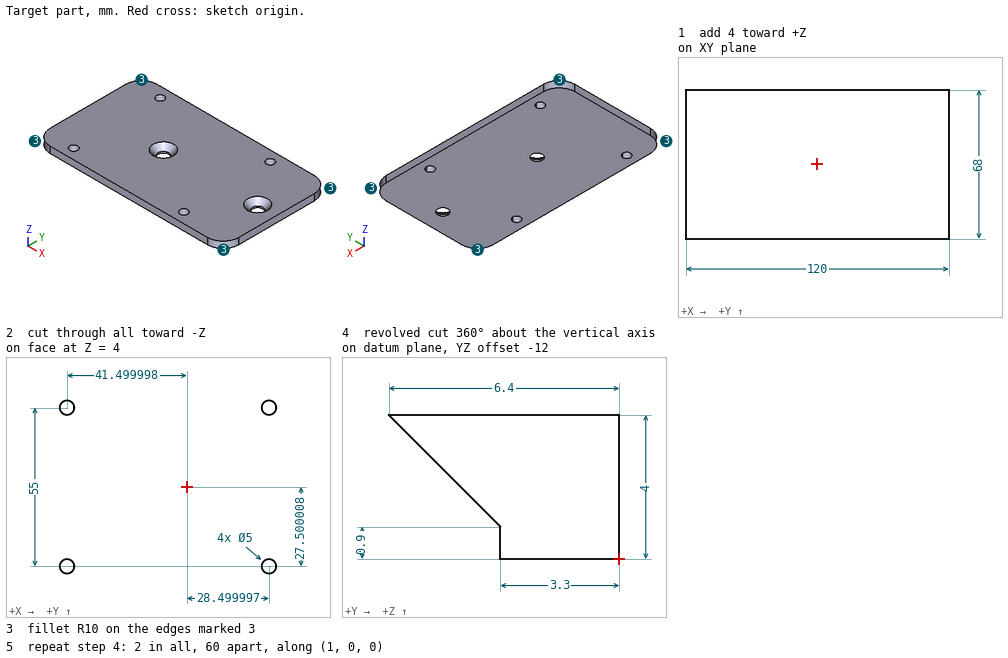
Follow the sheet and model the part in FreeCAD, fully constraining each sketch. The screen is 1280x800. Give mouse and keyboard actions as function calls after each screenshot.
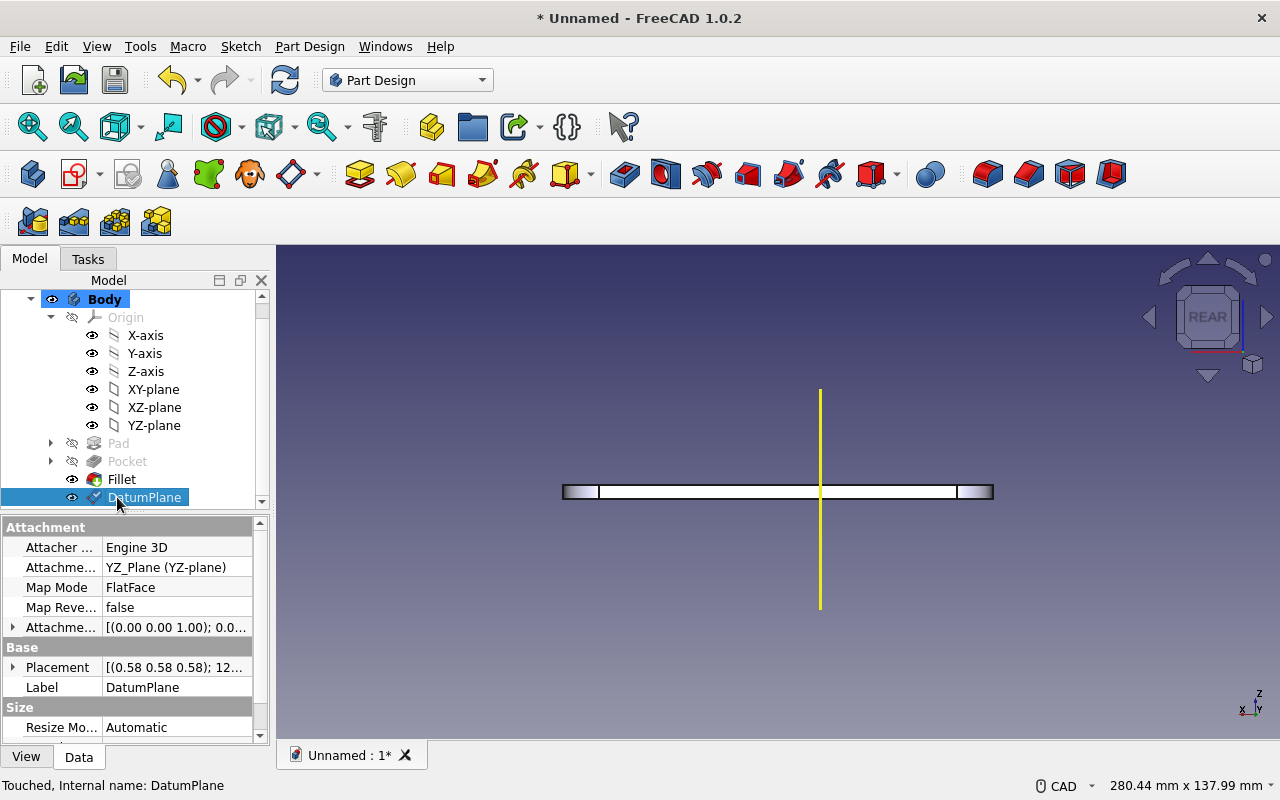
click(74, 174)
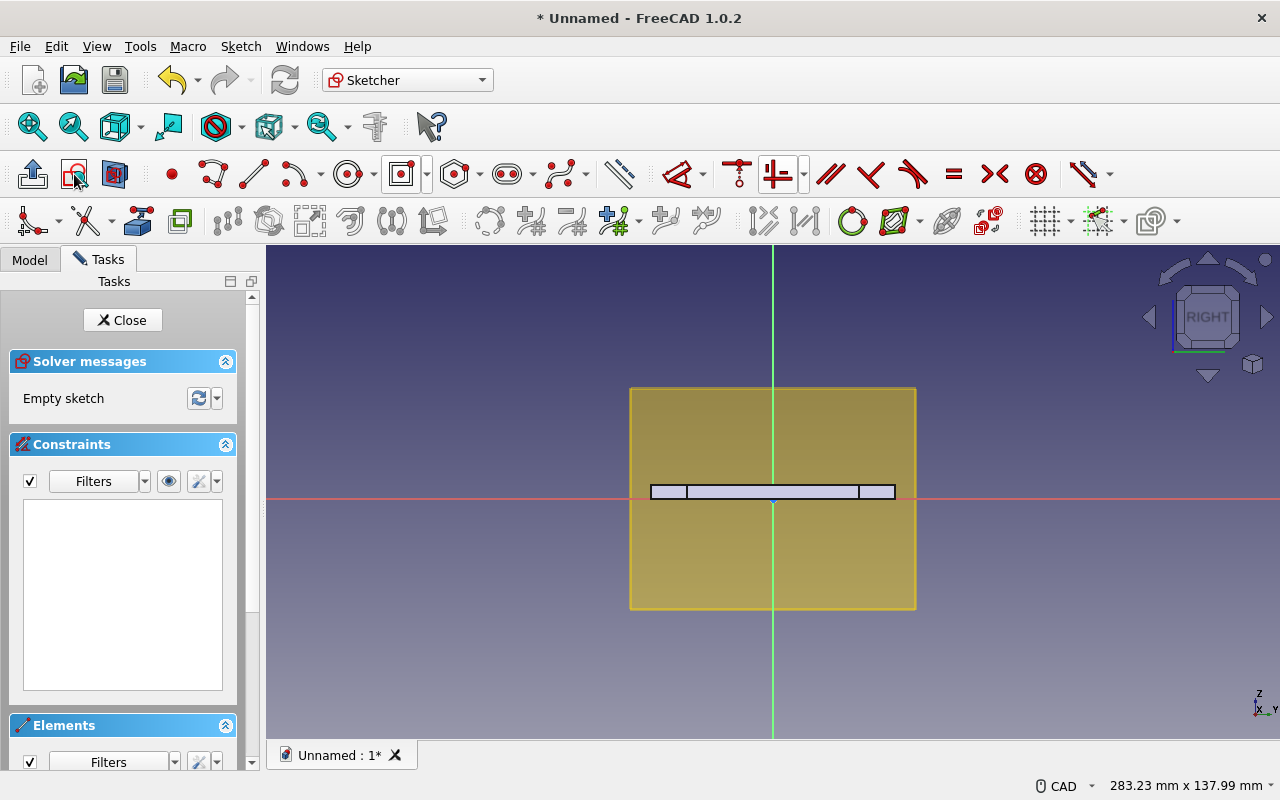
key(q)
key(s)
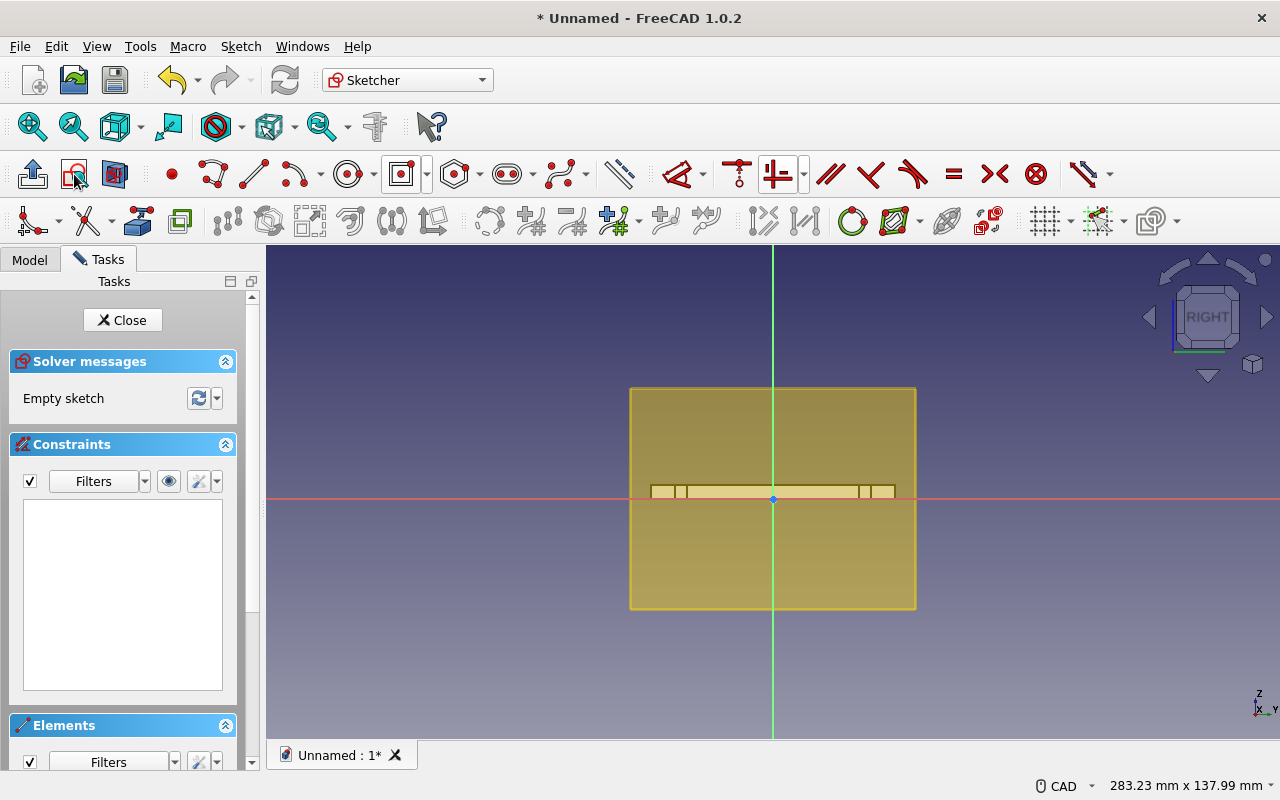
scroll(765, 492, up, 15)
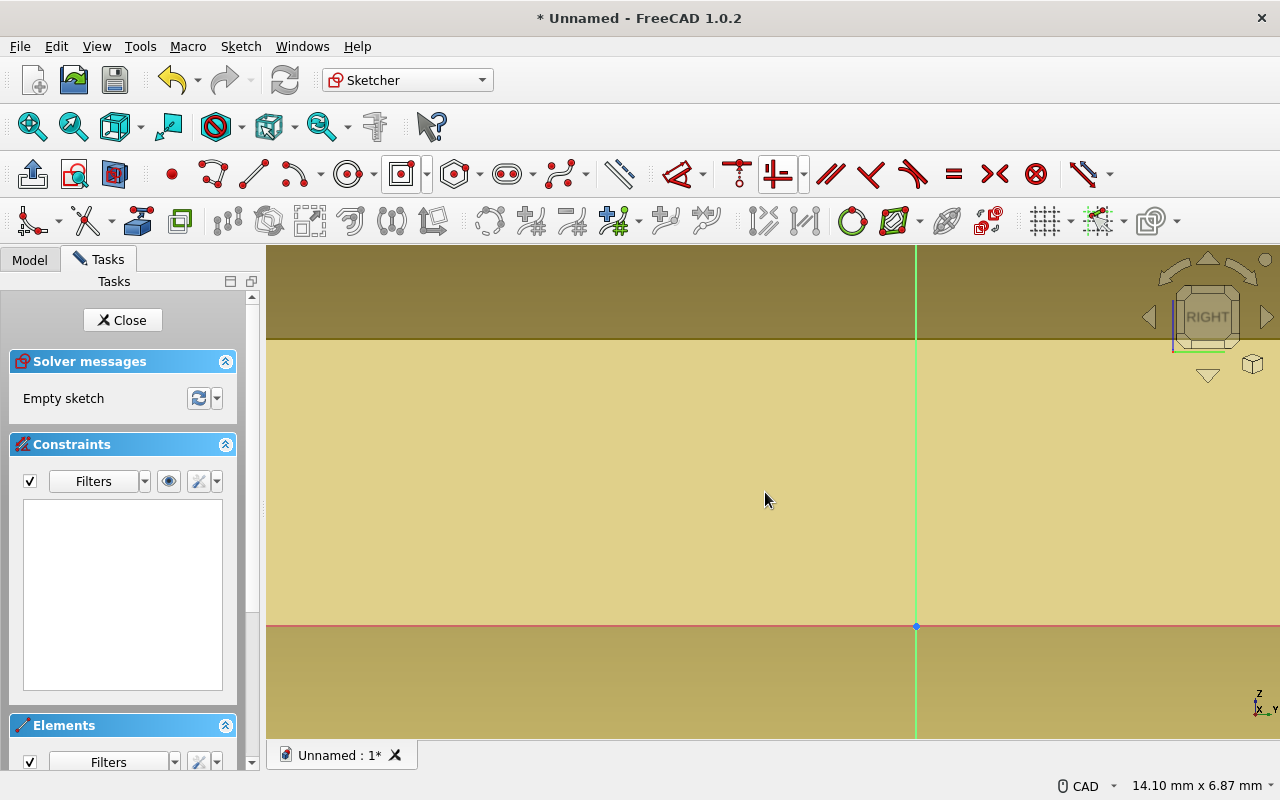
click(213, 174)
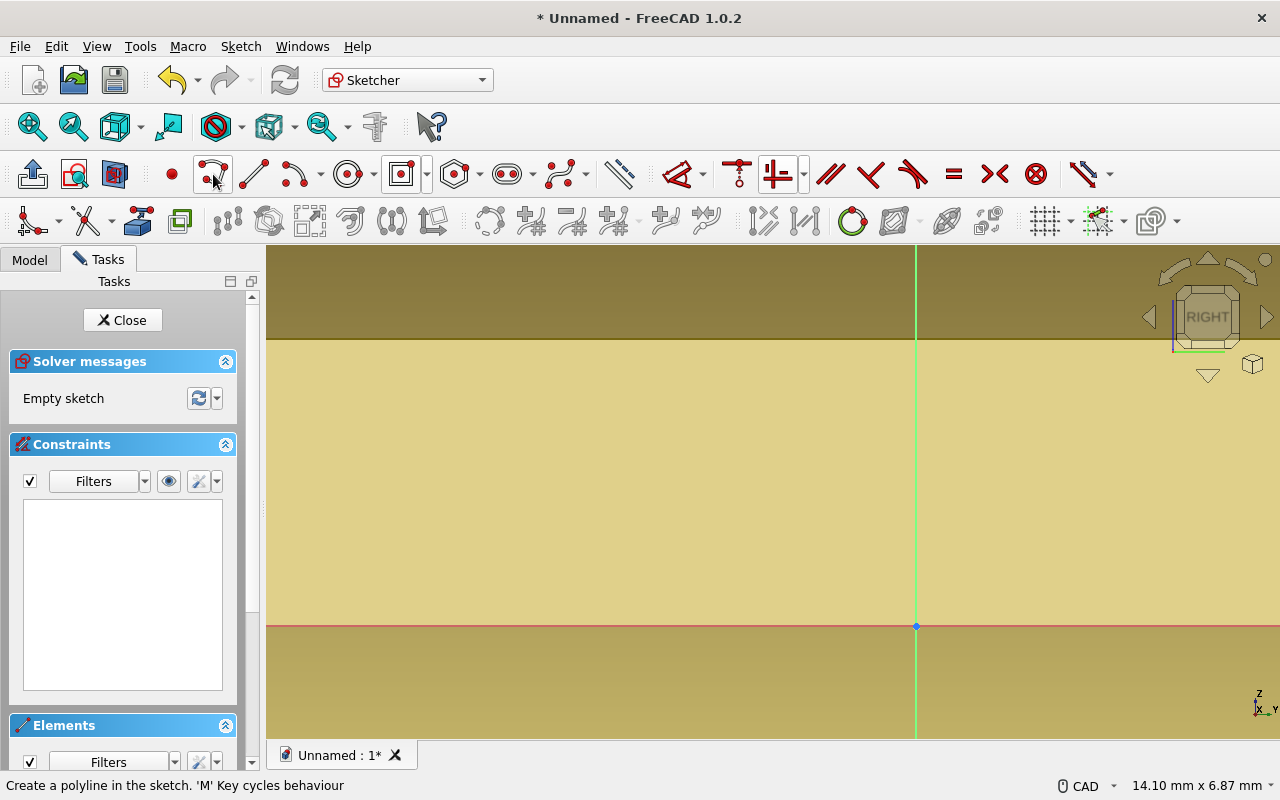
click(916, 626)
click(907, 339)
click(456, 339)
click(679, 562)
click(679, 617)
click(916, 626)
key(Escape)
key(Escape)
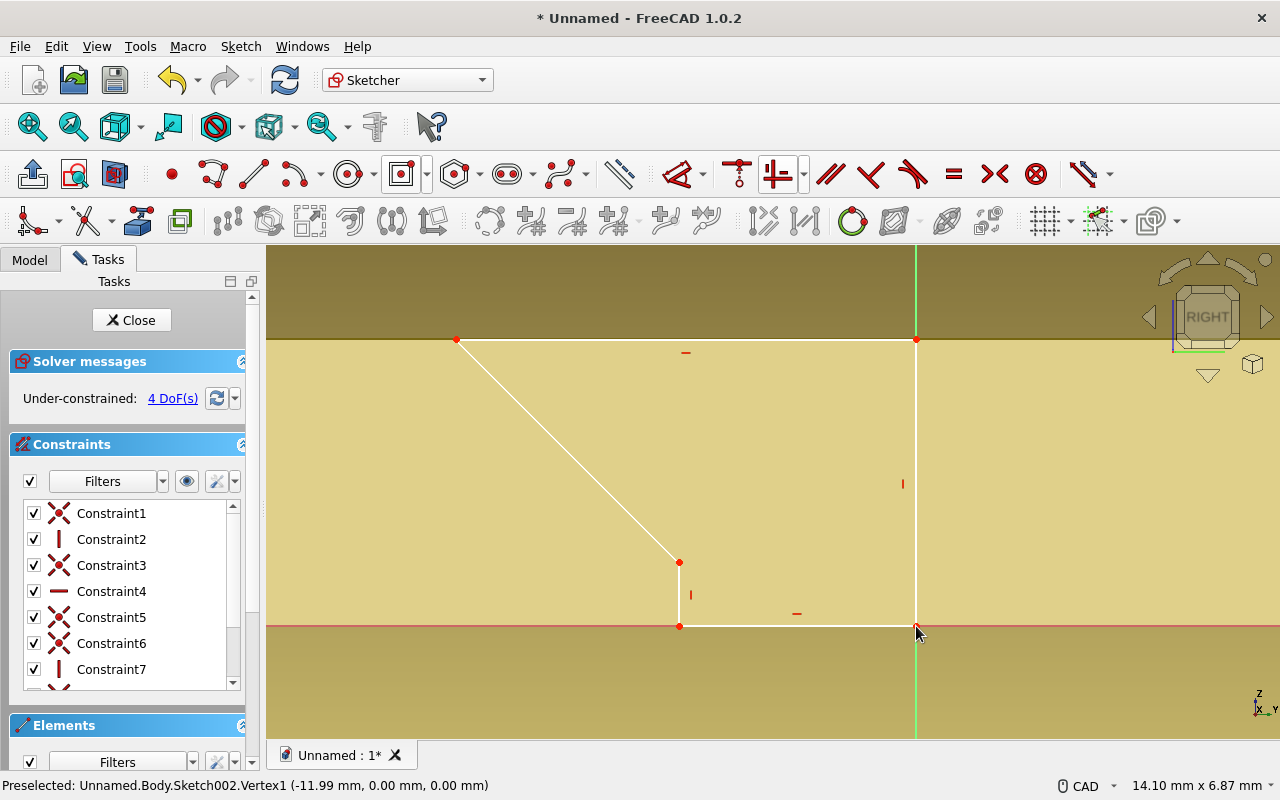
key(d)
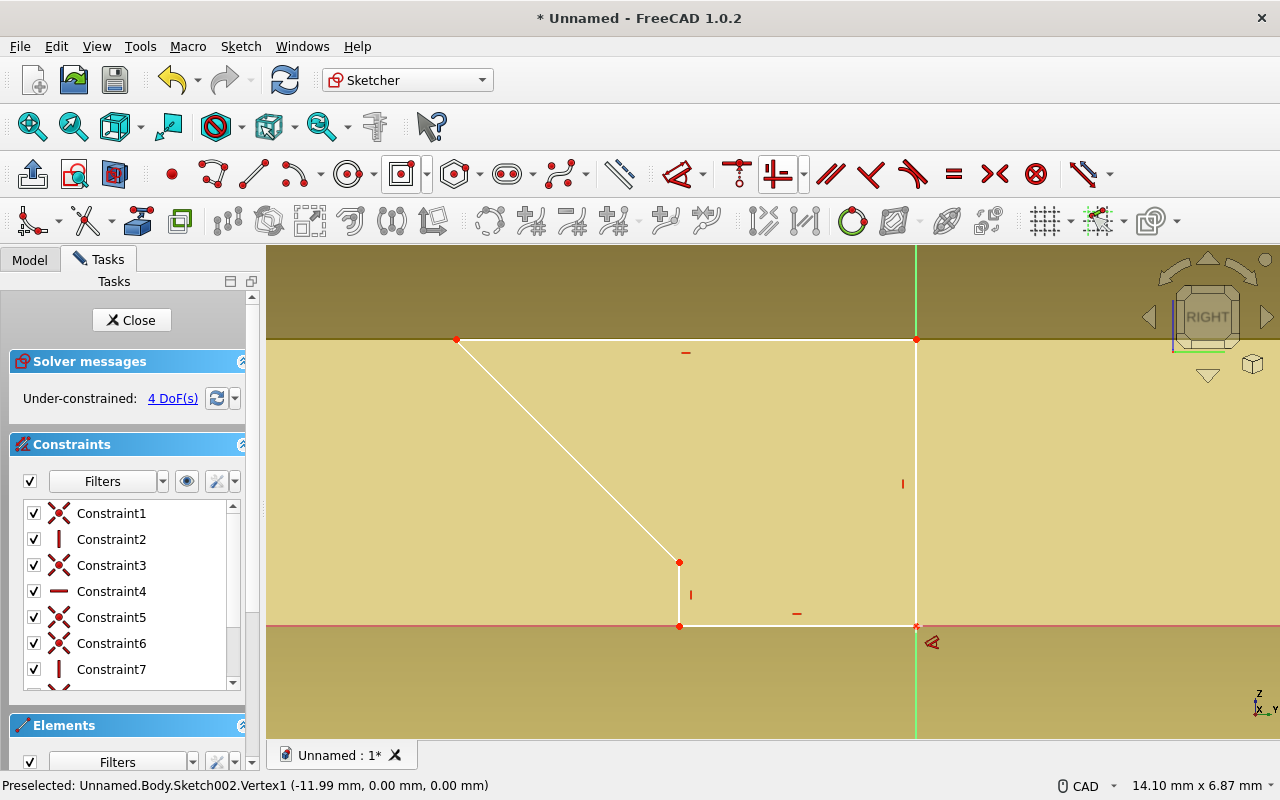
click(916, 540)
click(950, 483)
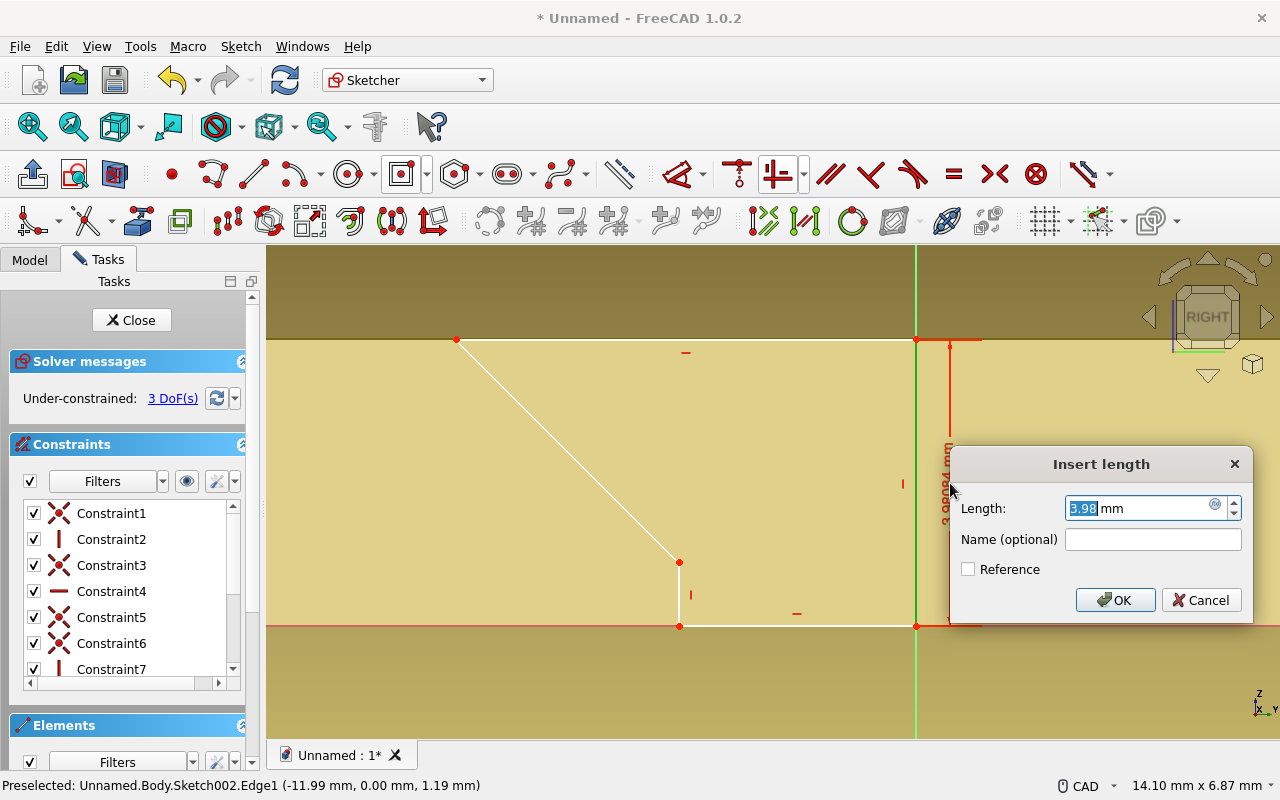
text(4)
key(Return)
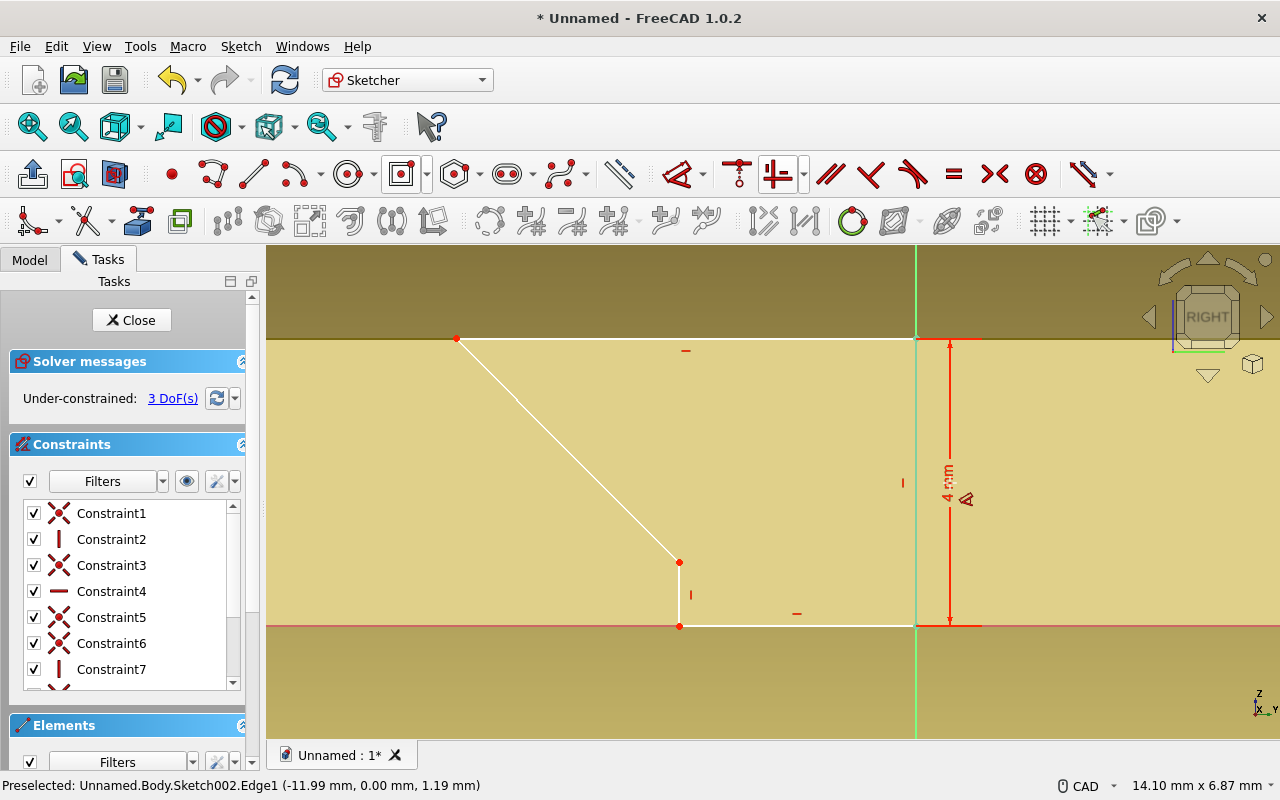
click(778, 339)
click(686, 305)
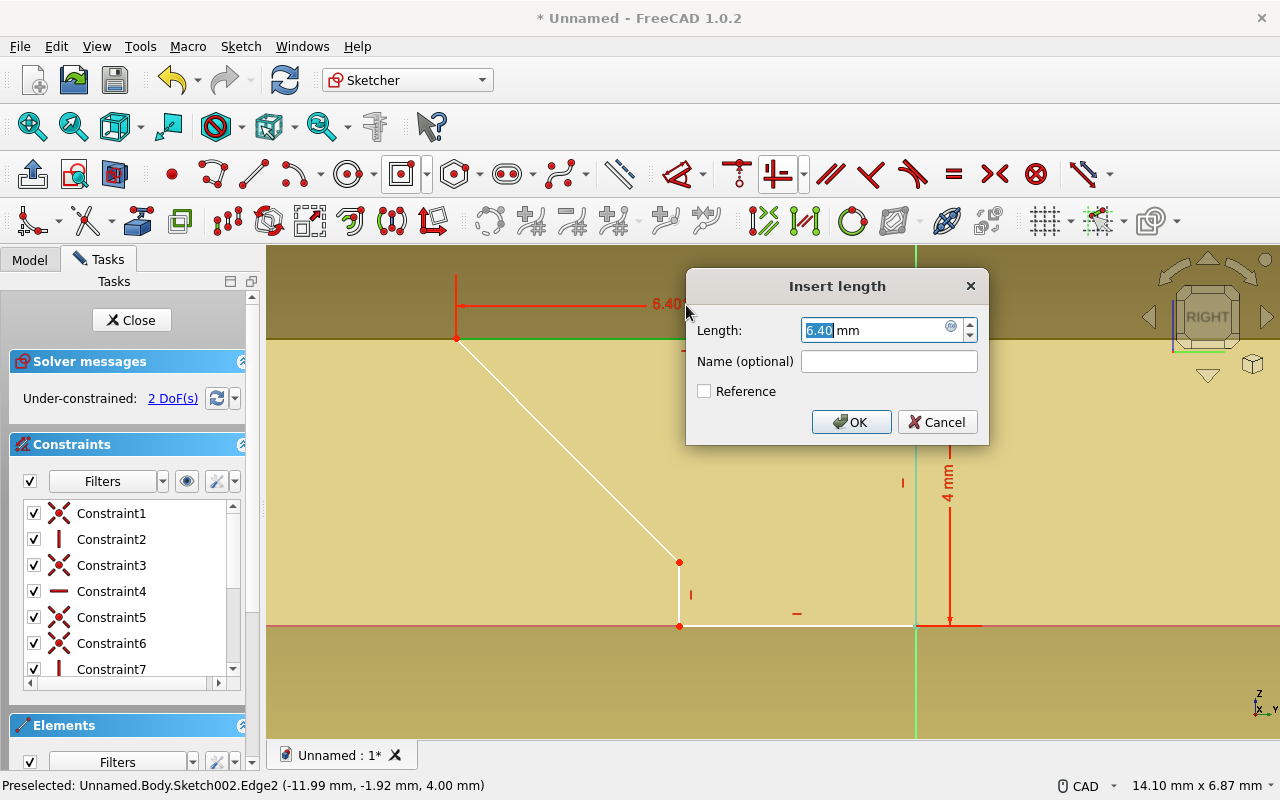
text(6.4)
key(Return)